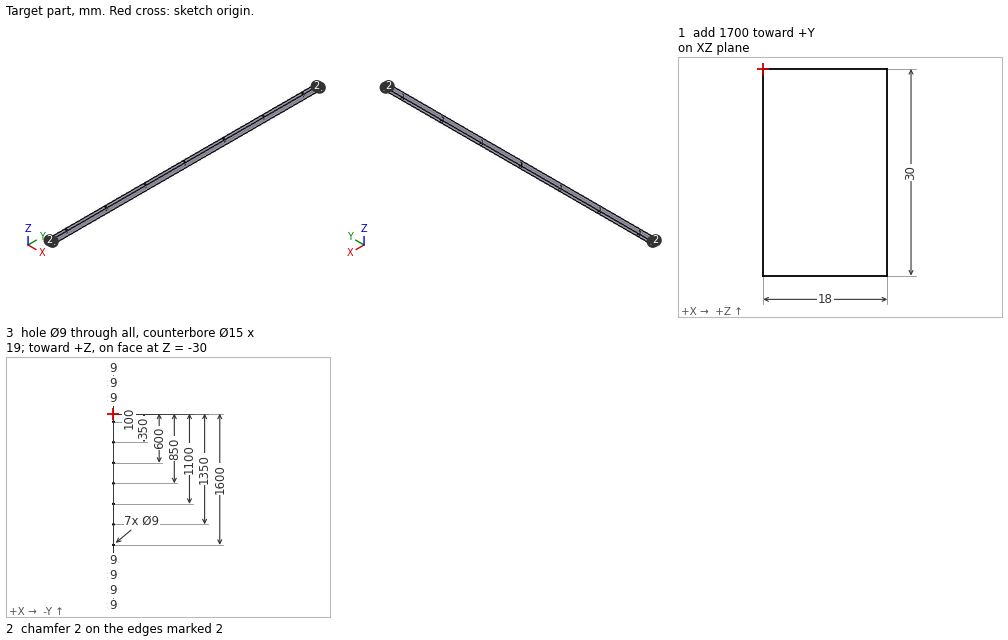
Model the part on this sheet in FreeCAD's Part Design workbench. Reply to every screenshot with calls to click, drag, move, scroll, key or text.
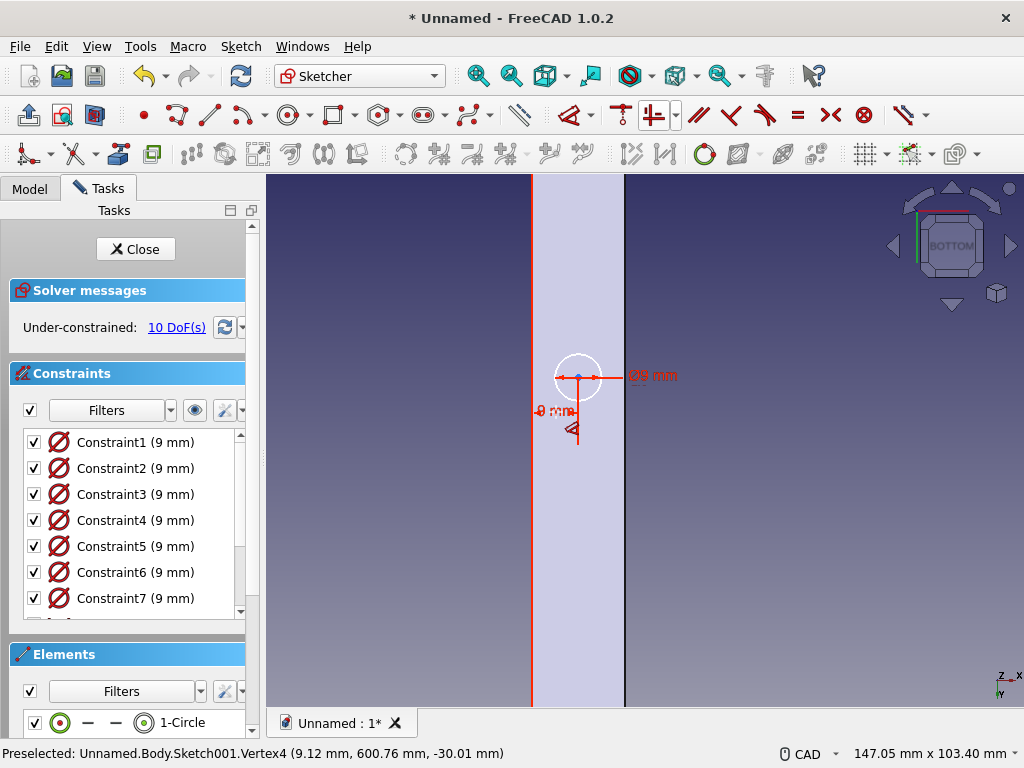
scroll(577, 389, down, 15)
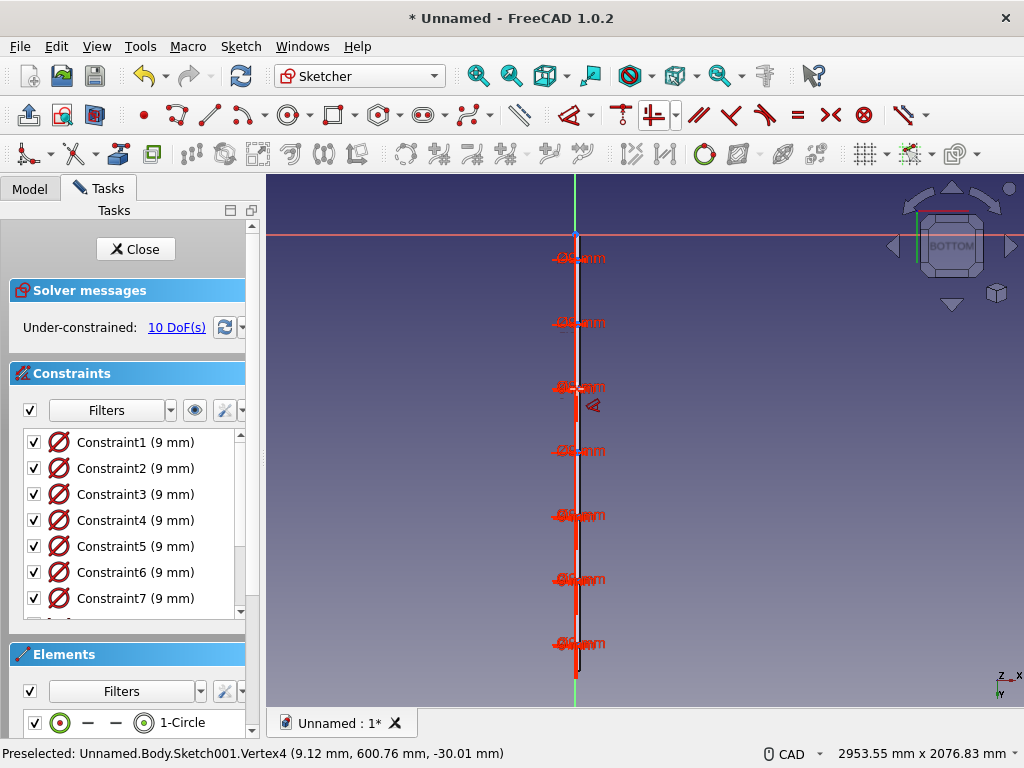
scroll(577, 325, up, 15)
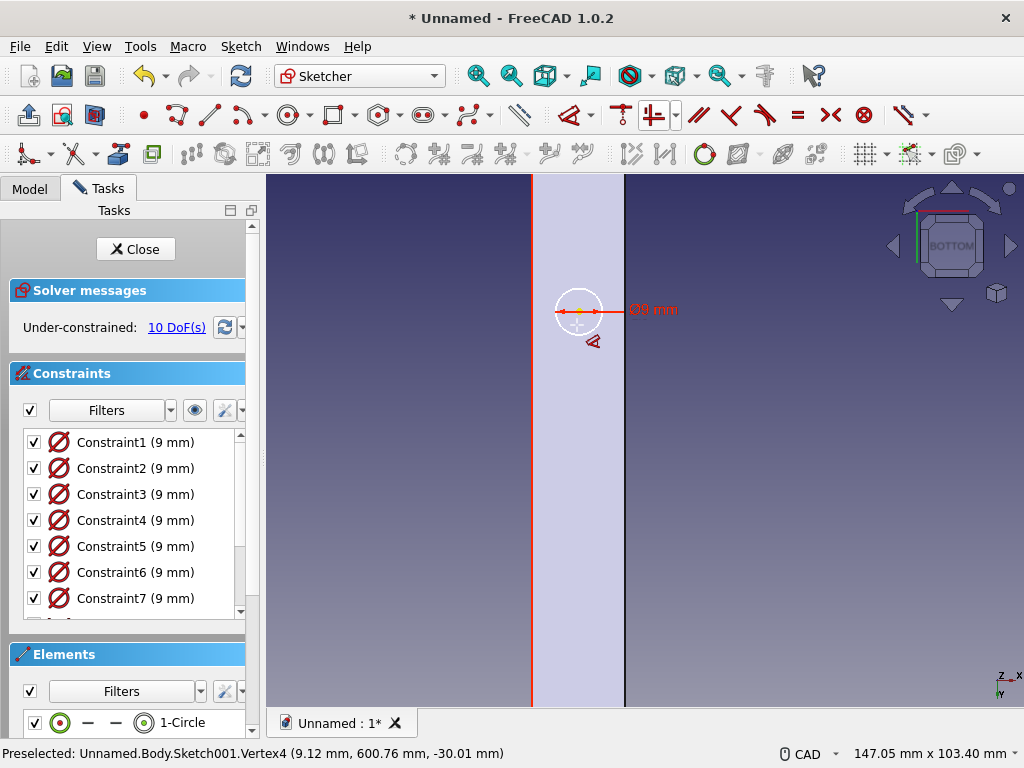
click(579, 312)
click(556, 346)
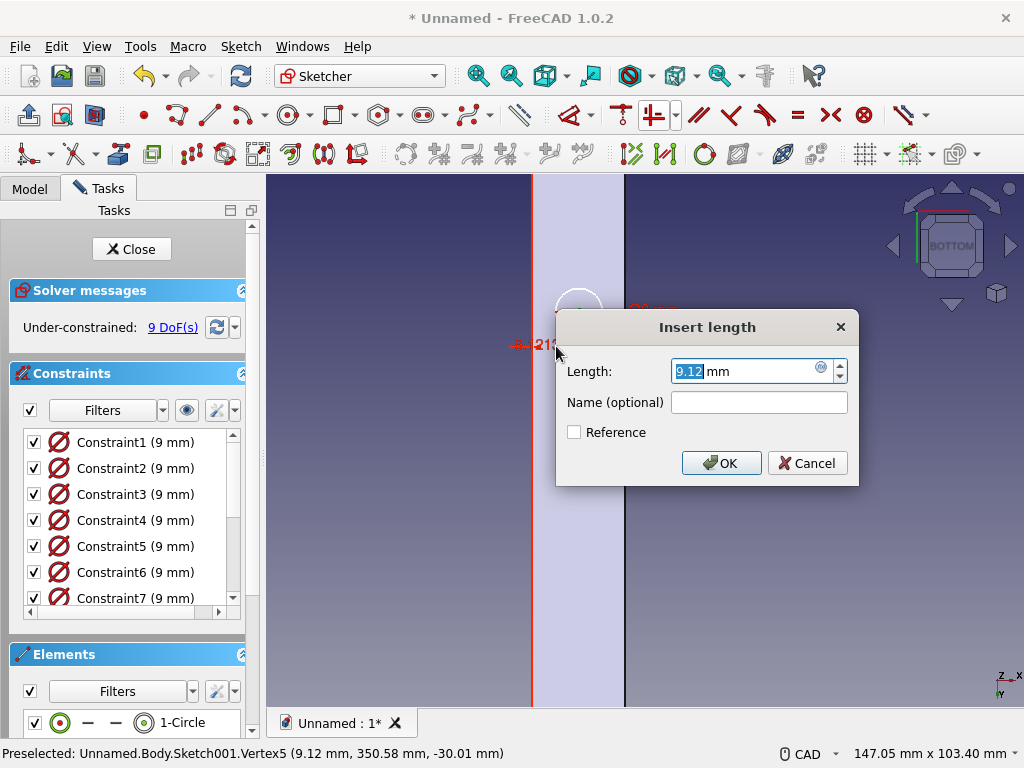
text(9)
key(Return)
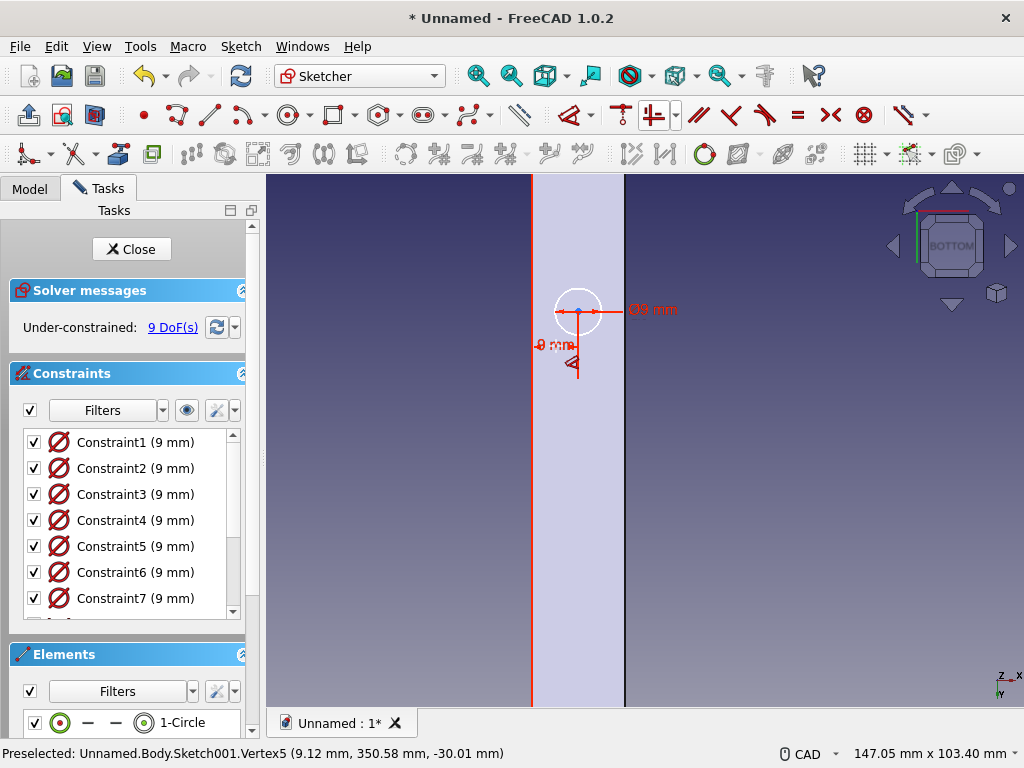
scroll(577, 325, down, 15)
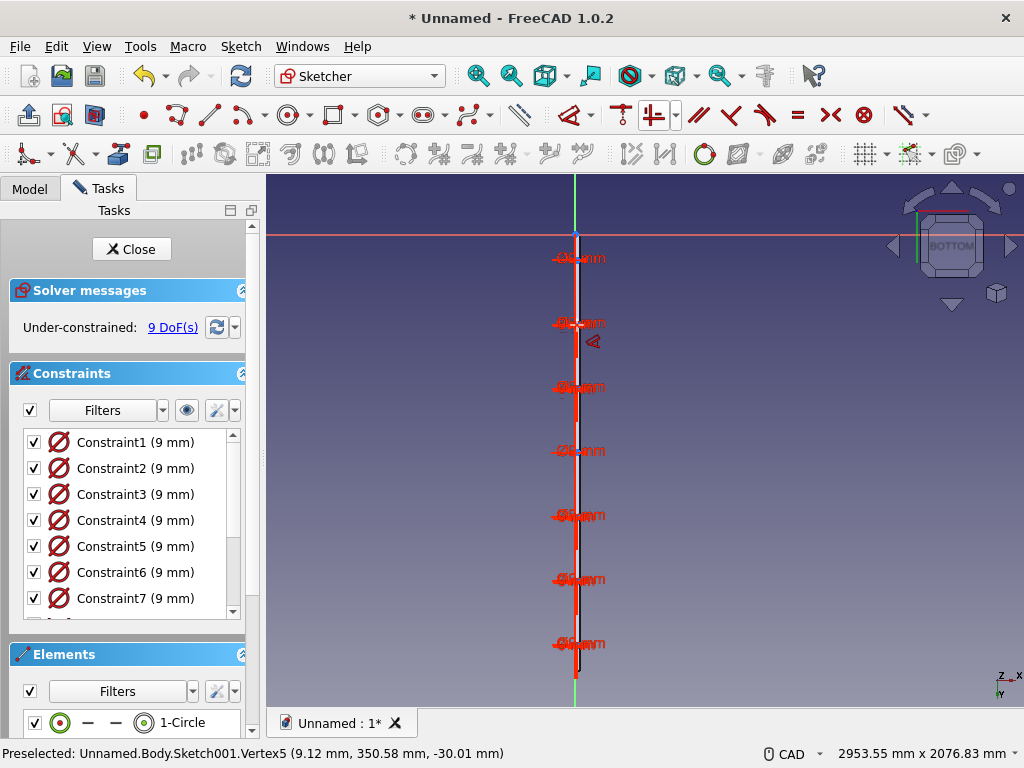
scroll(577, 260, up, 15)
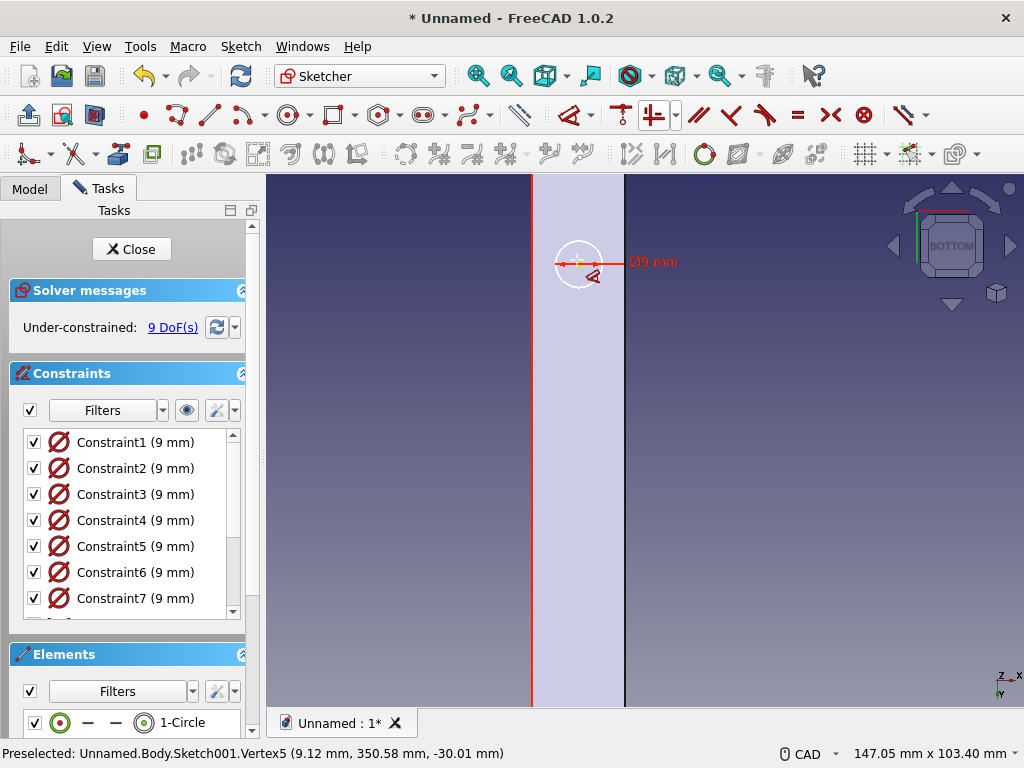
click(579, 264)
click(556, 298)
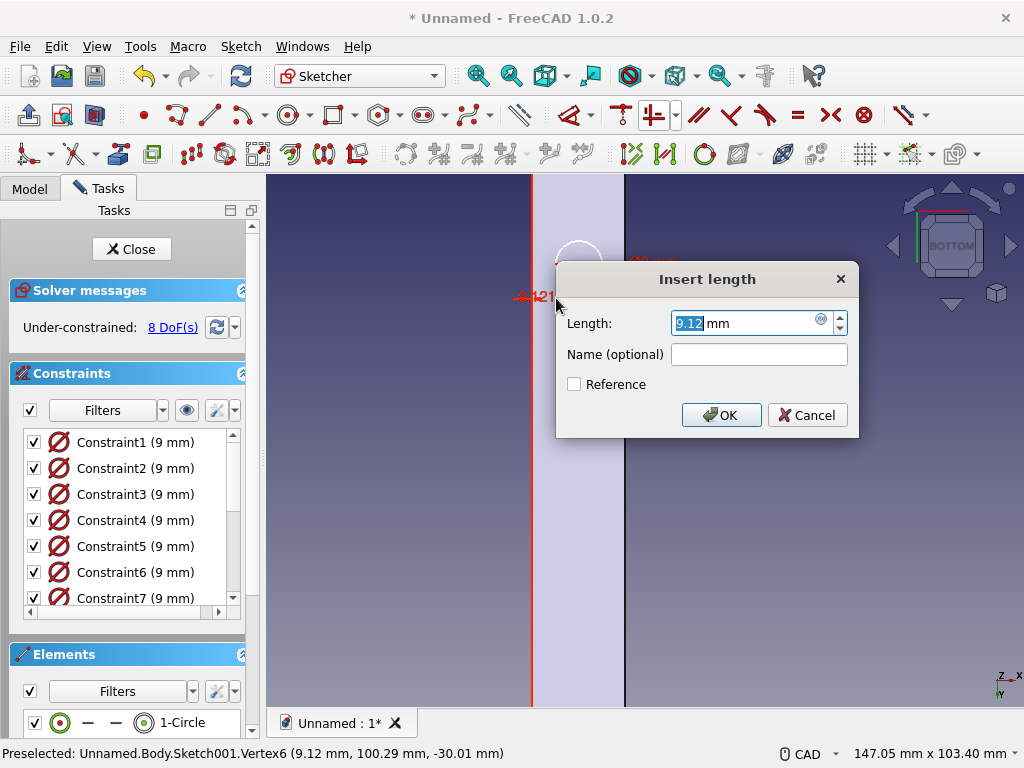
text(9)
key(Return)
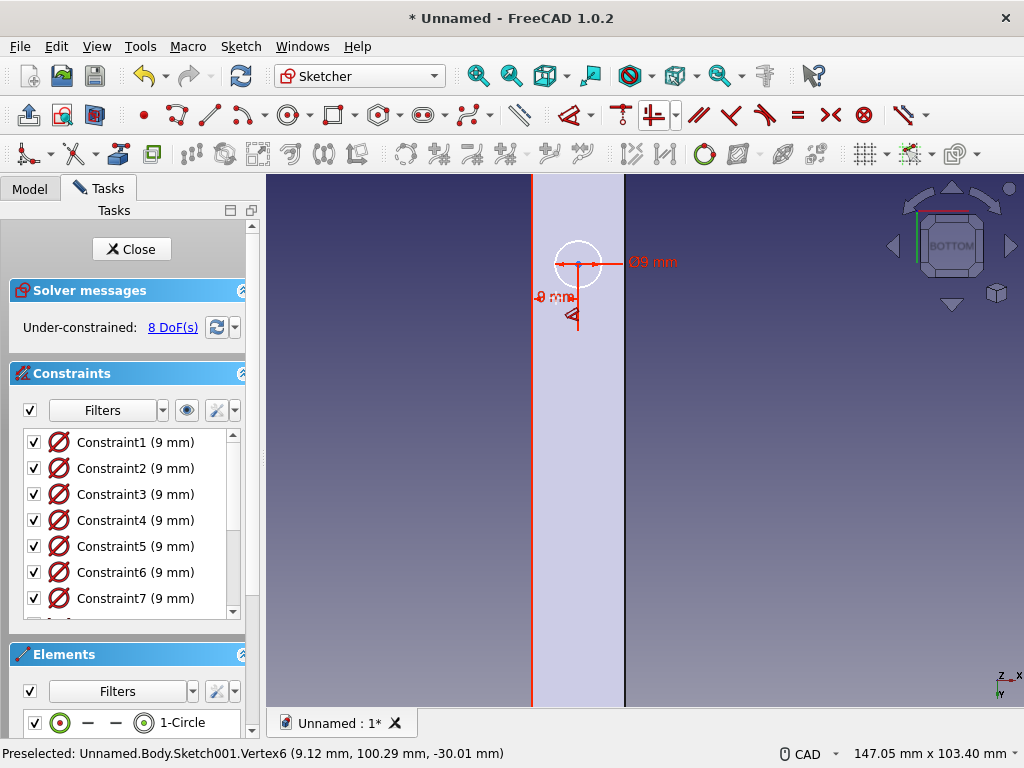
scroll(577, 260, down, 15)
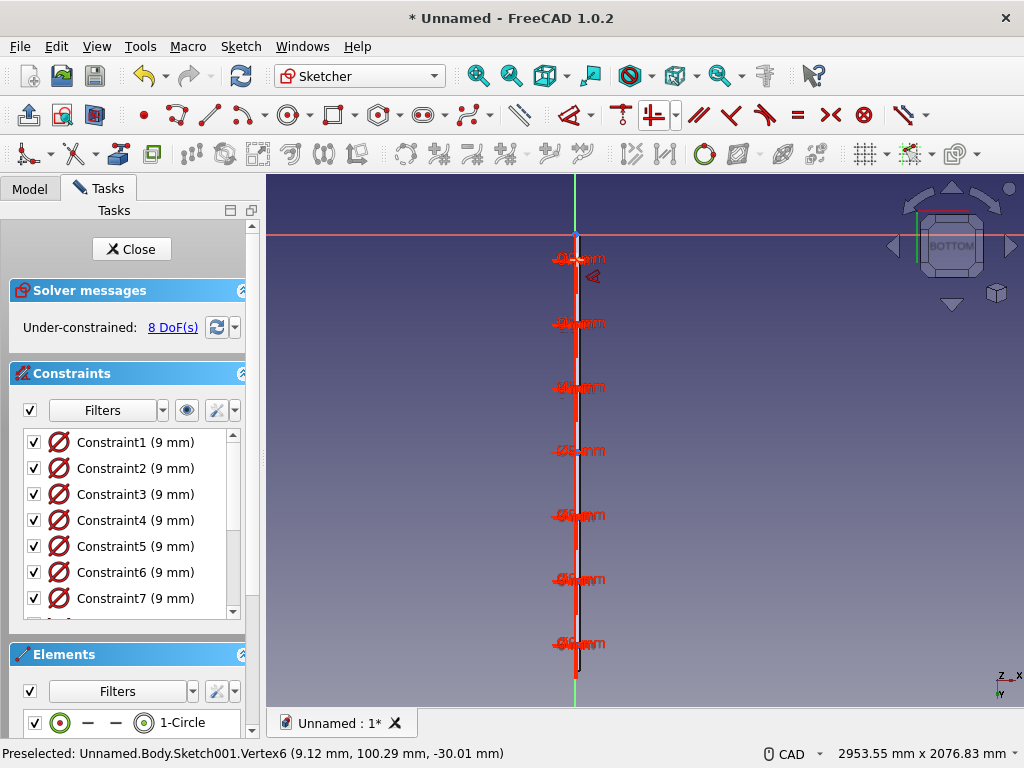
scroll(577, 453, up, 15)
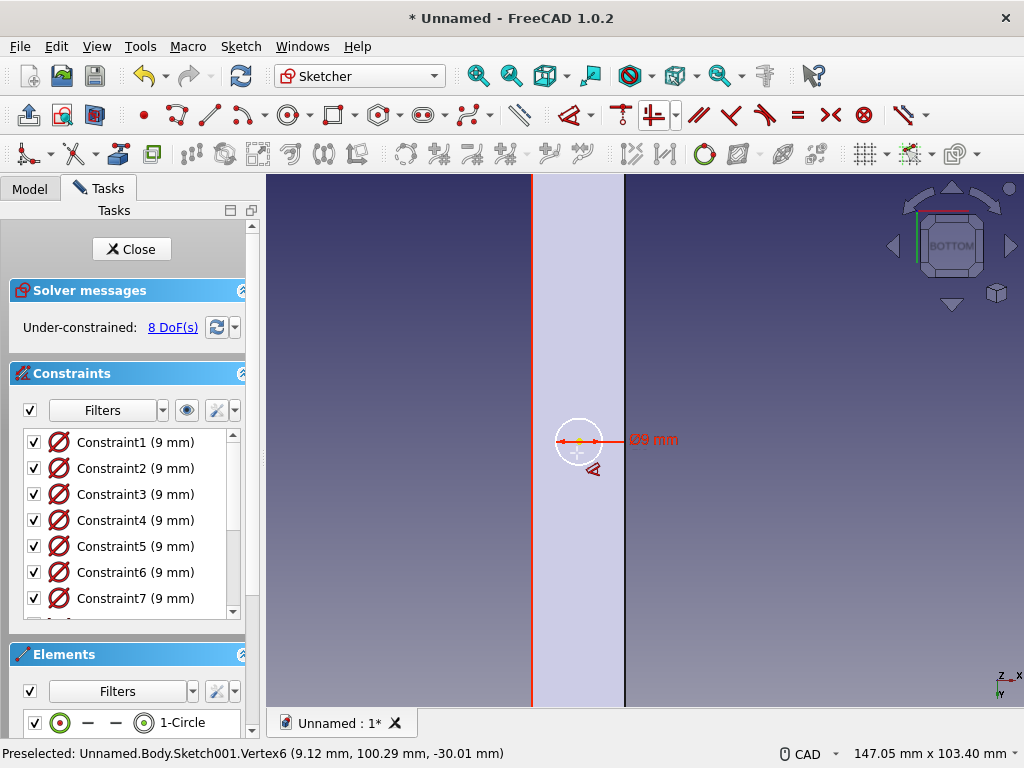
click(579, 442)
click(556, 476)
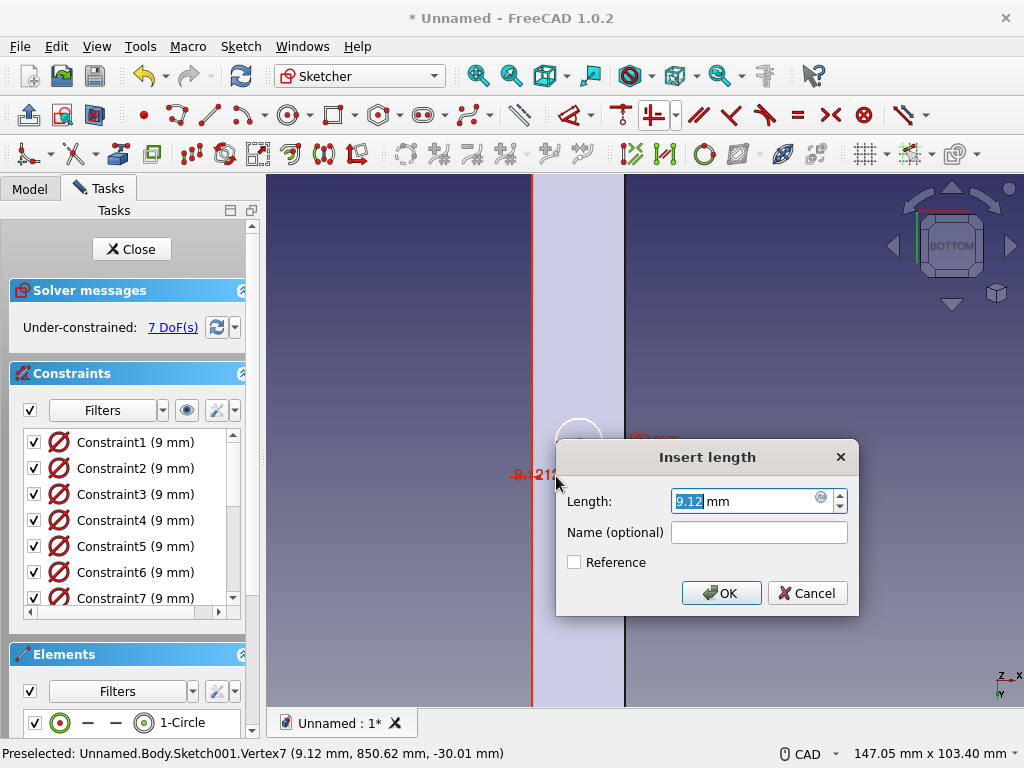
text(9)
key(Return)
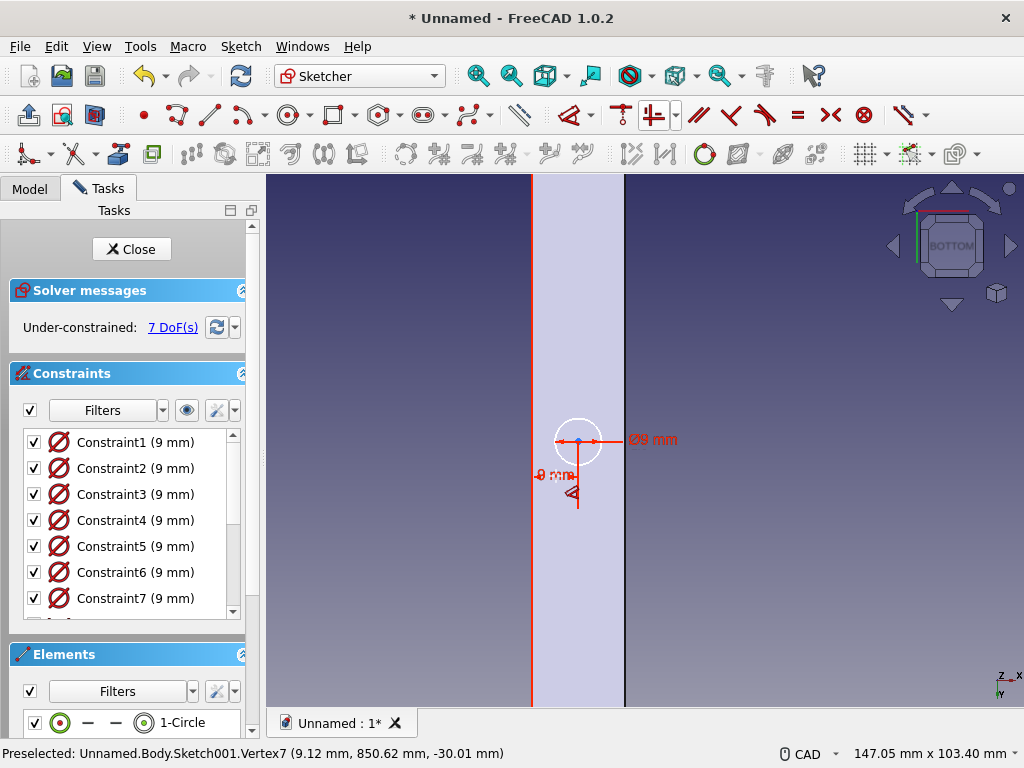
scroll(577, 454, down, 15)